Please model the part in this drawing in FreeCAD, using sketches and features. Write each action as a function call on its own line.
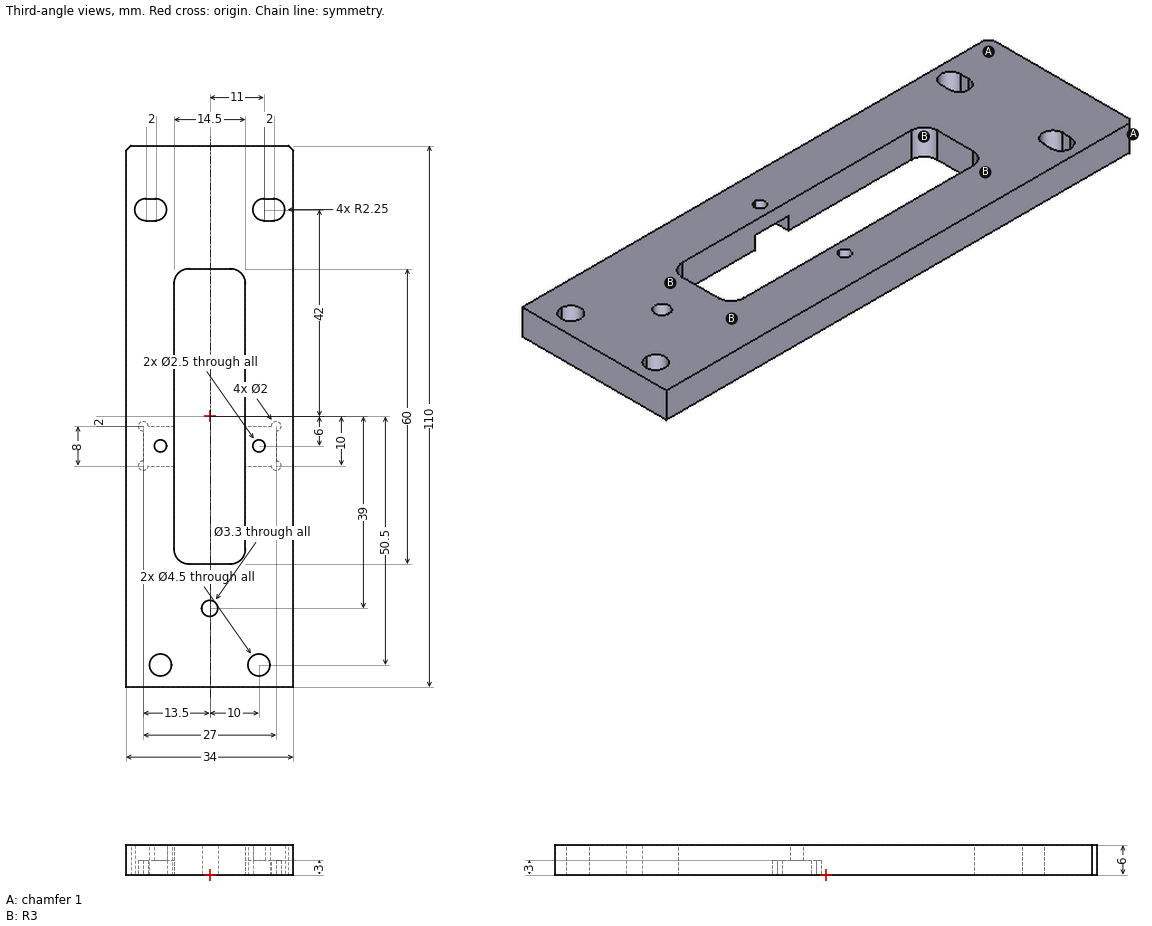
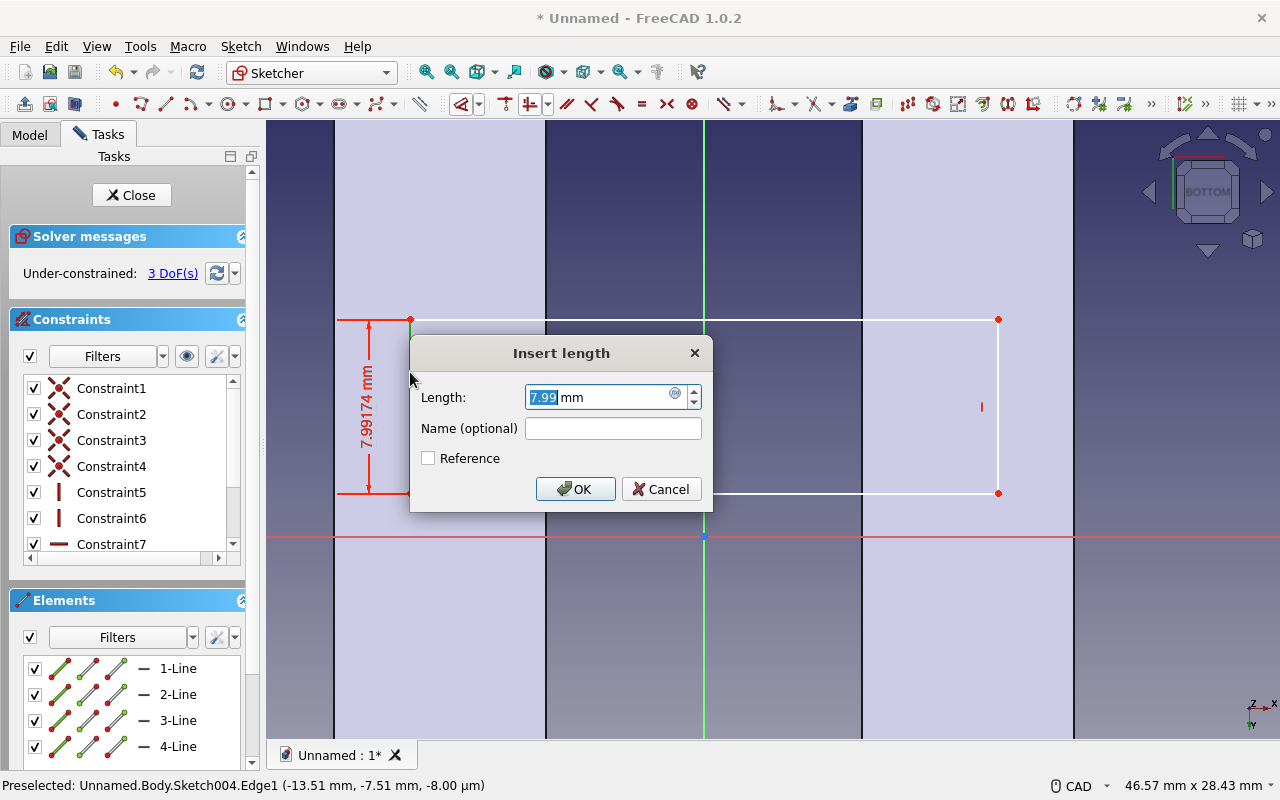
text(8)
key(Return)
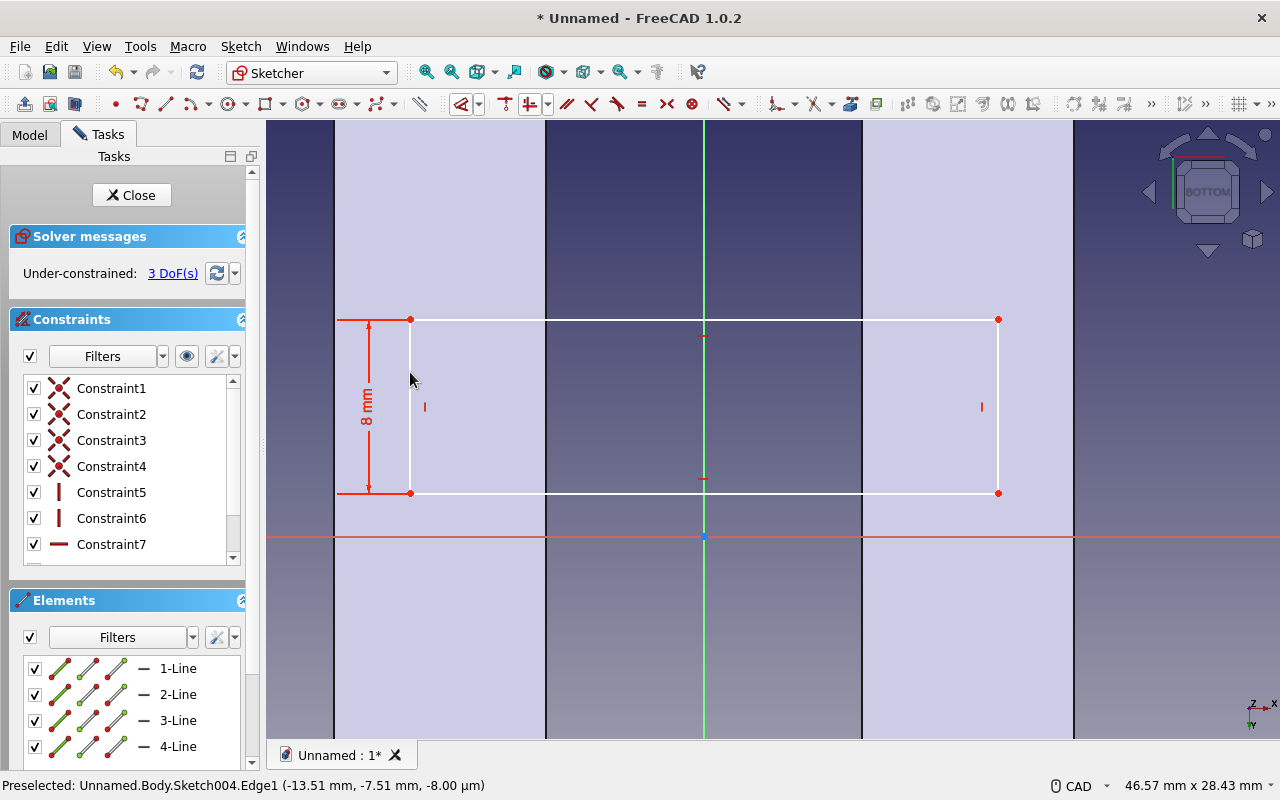
click(586, 494)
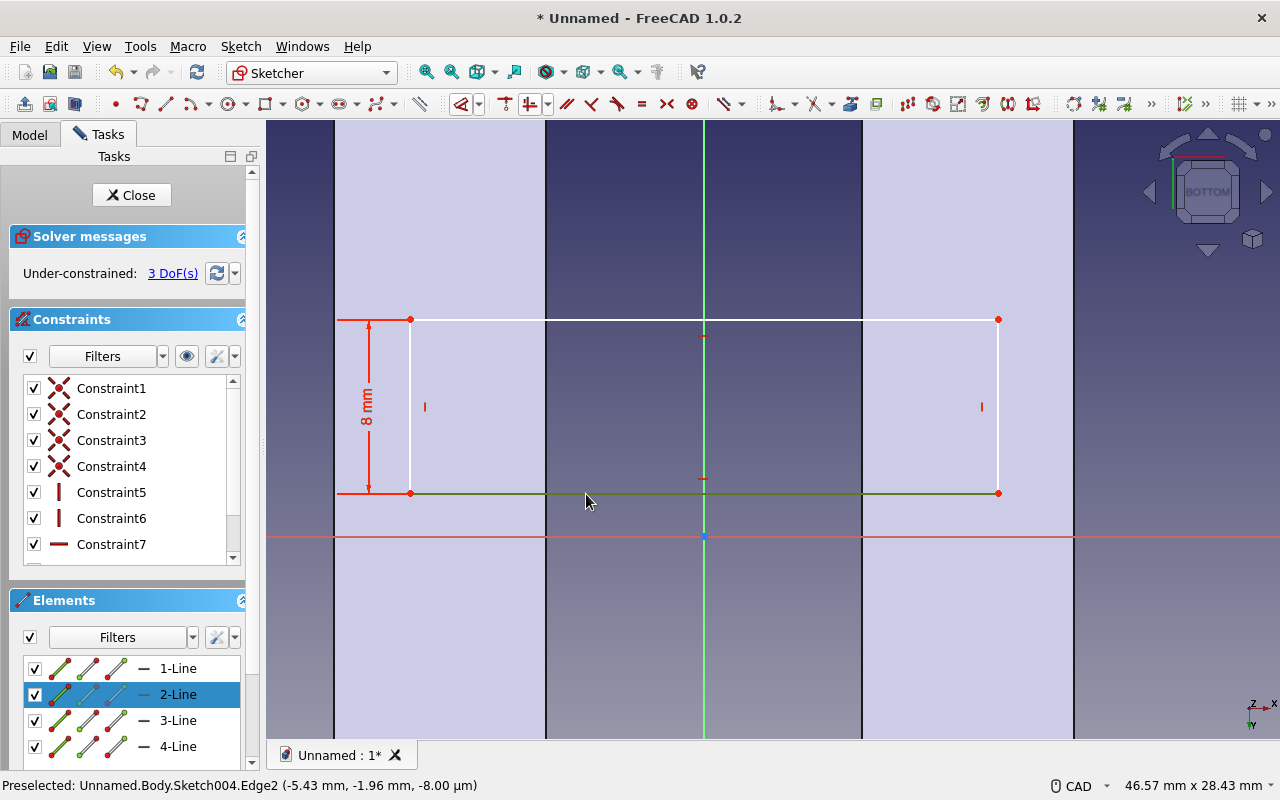
click(478, 104)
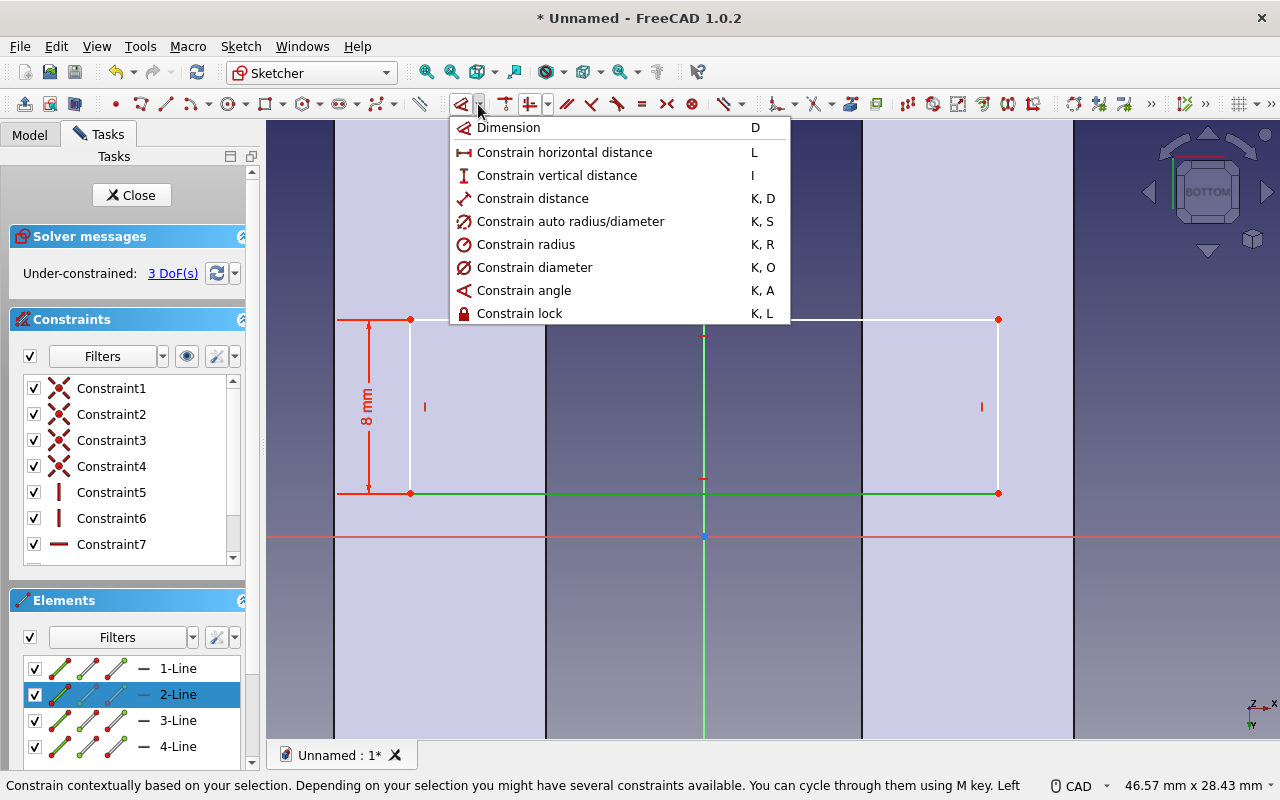
click(620, 152)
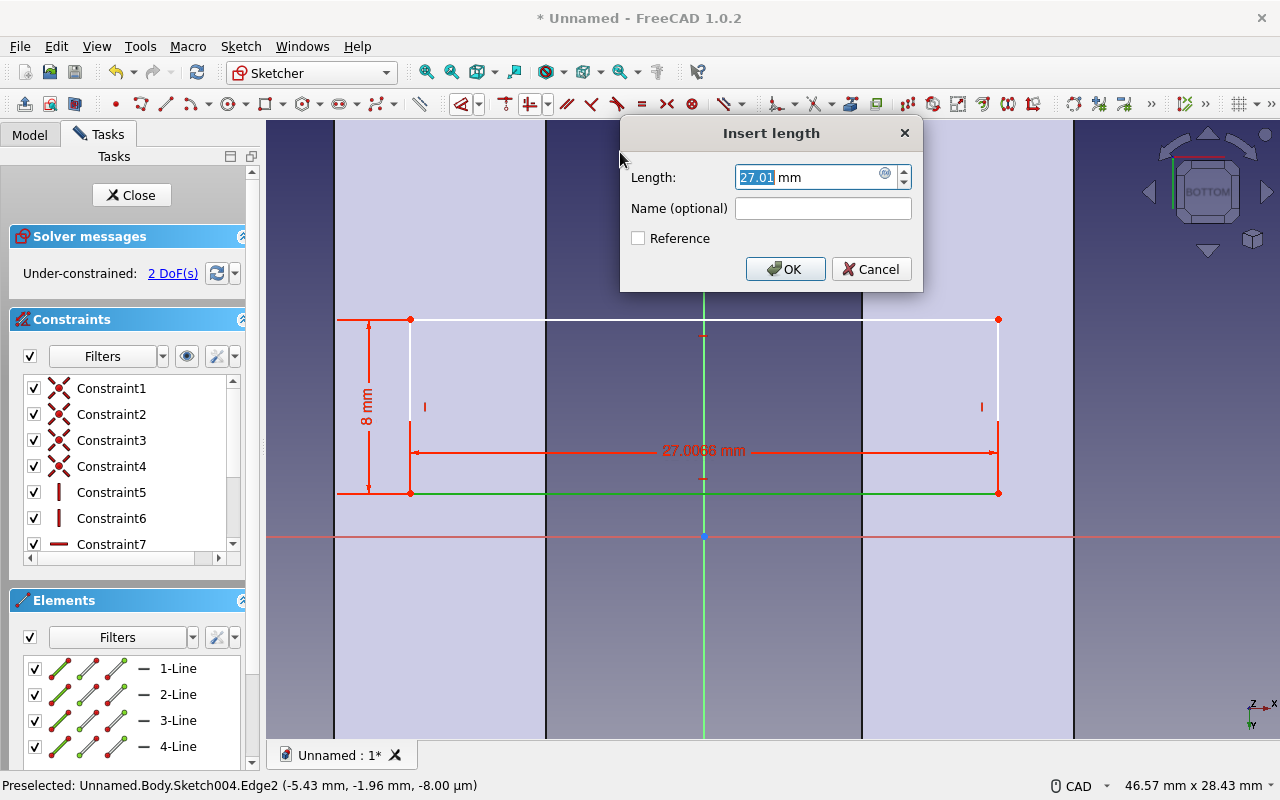
text(27)
key(Return)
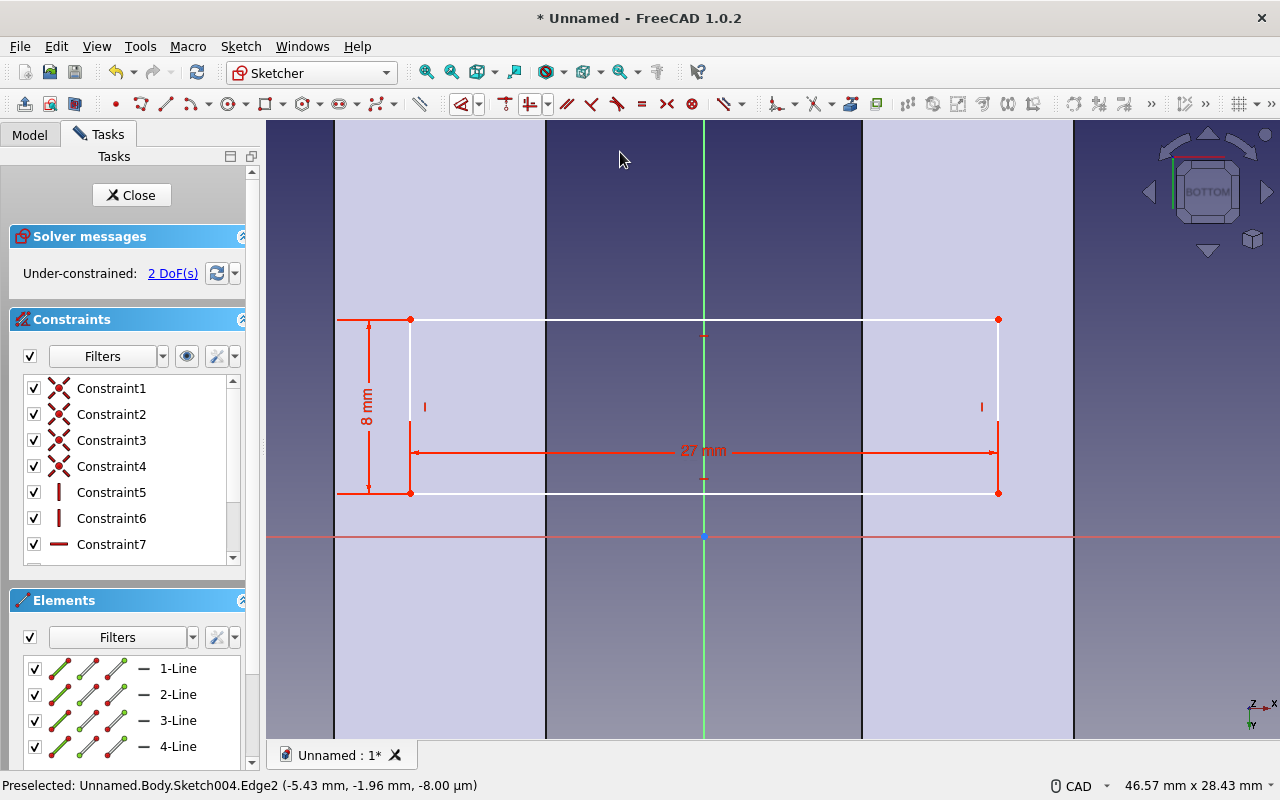
click(410, 494)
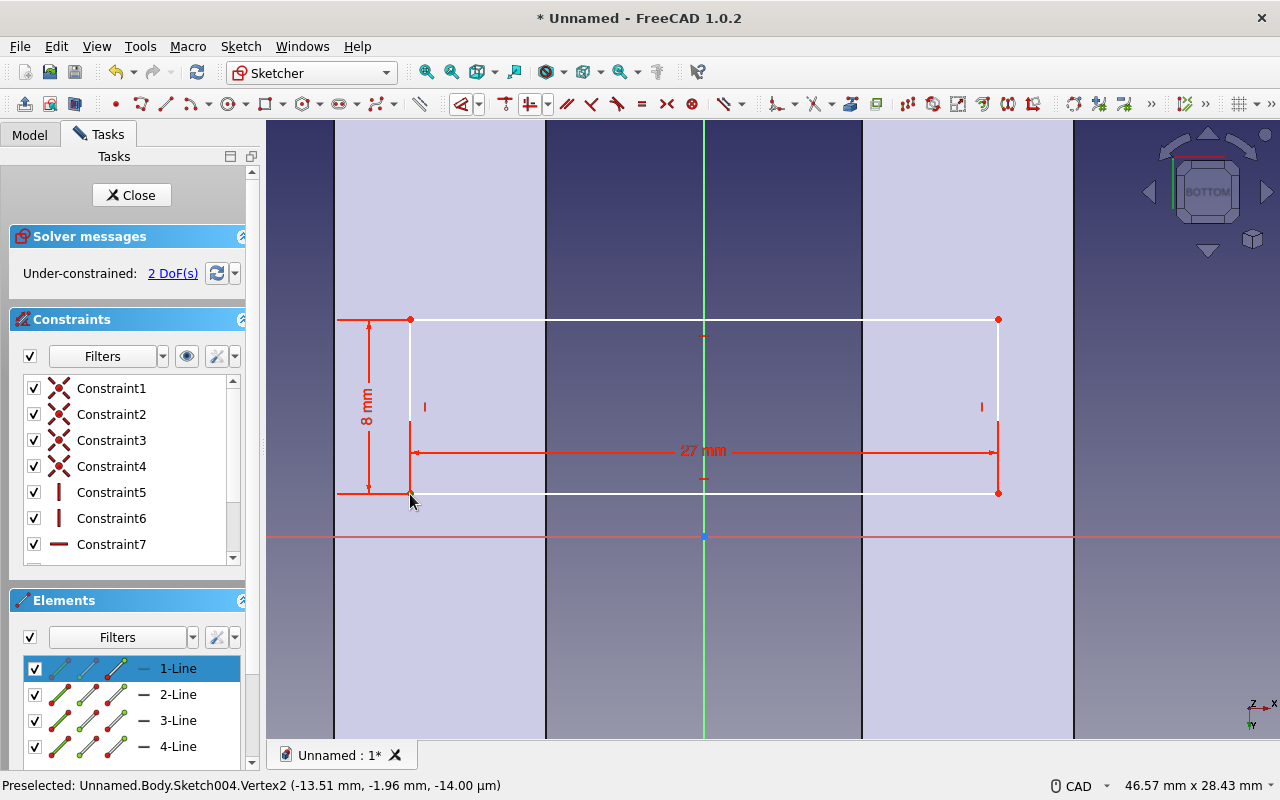
key(i)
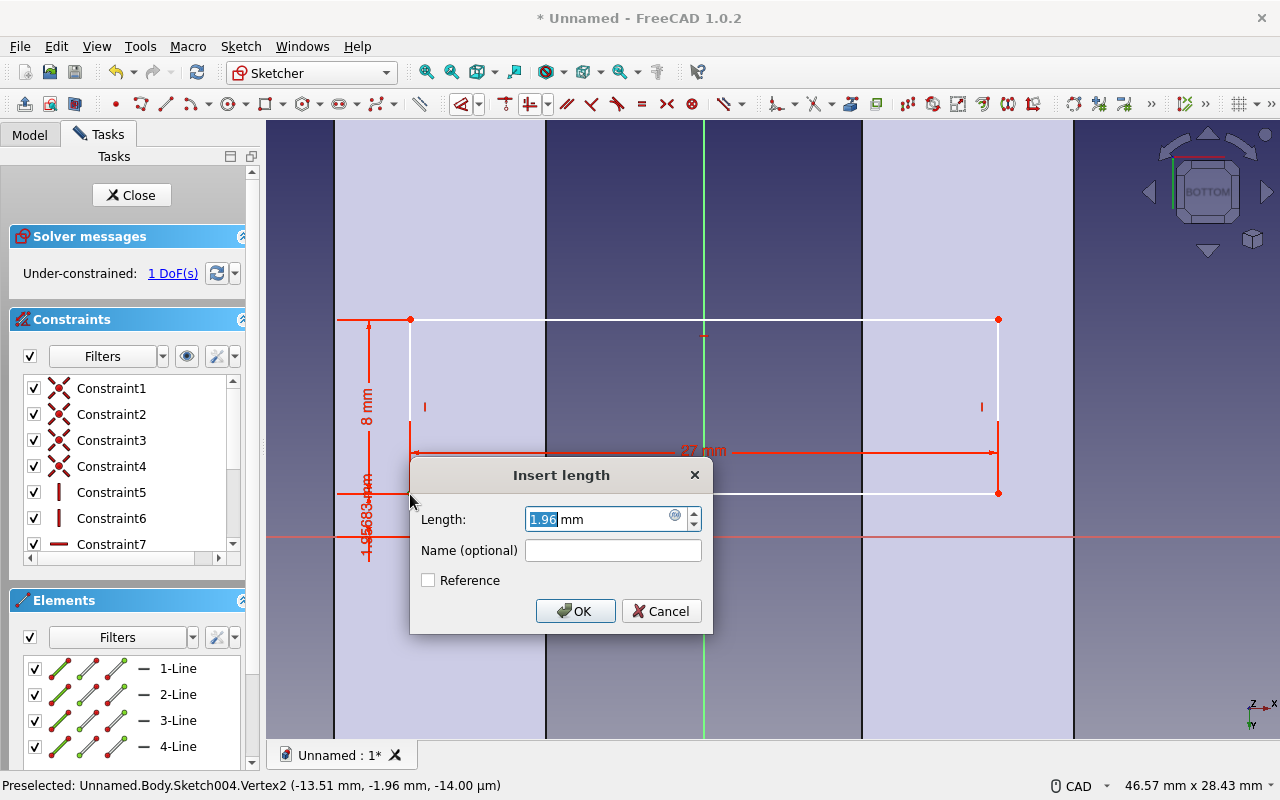
text(2)
key(Return)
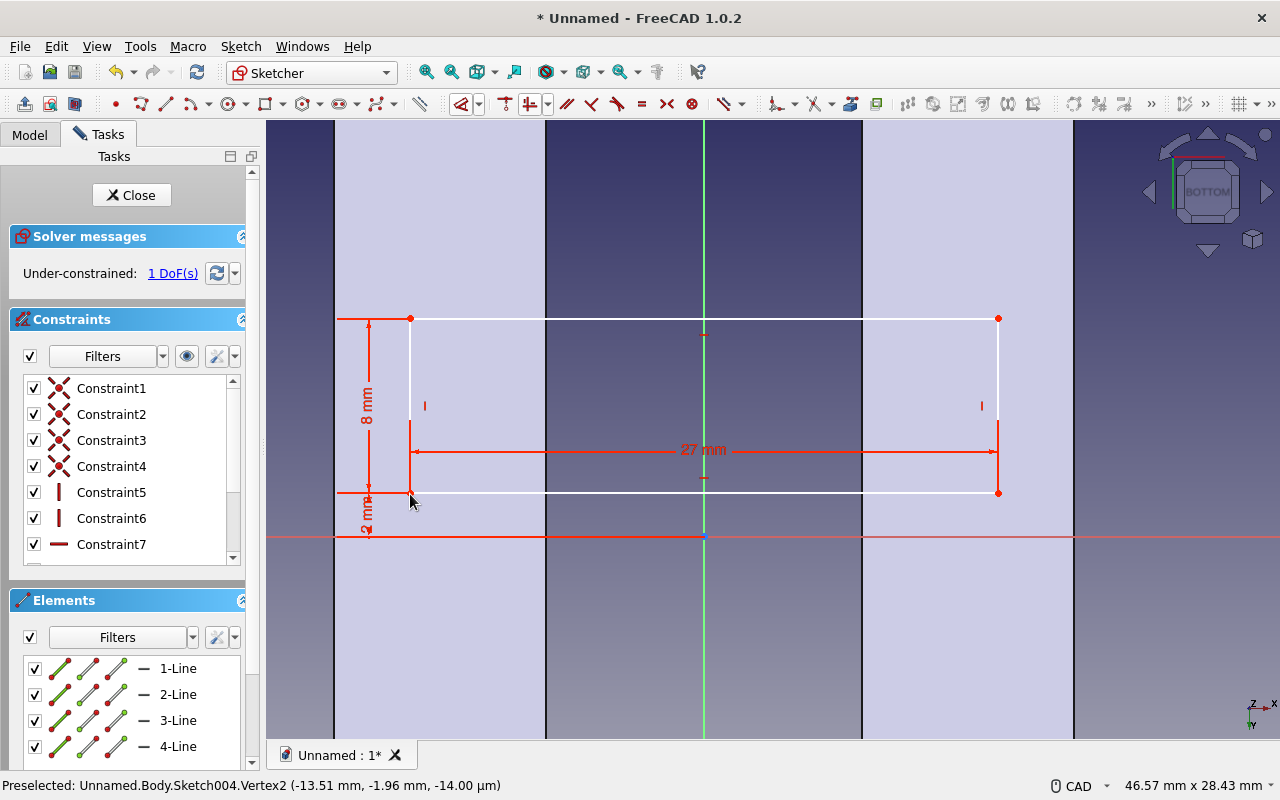
click(410, 319)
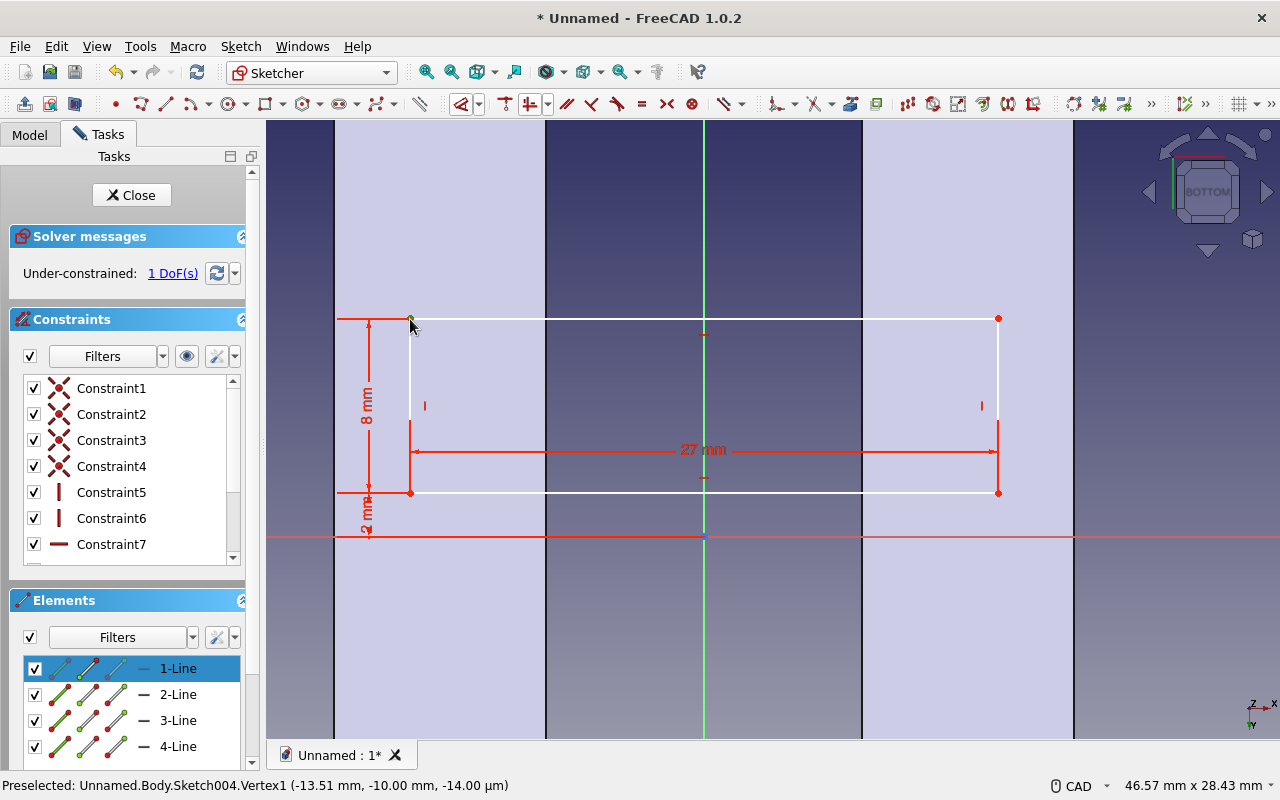
key(l)